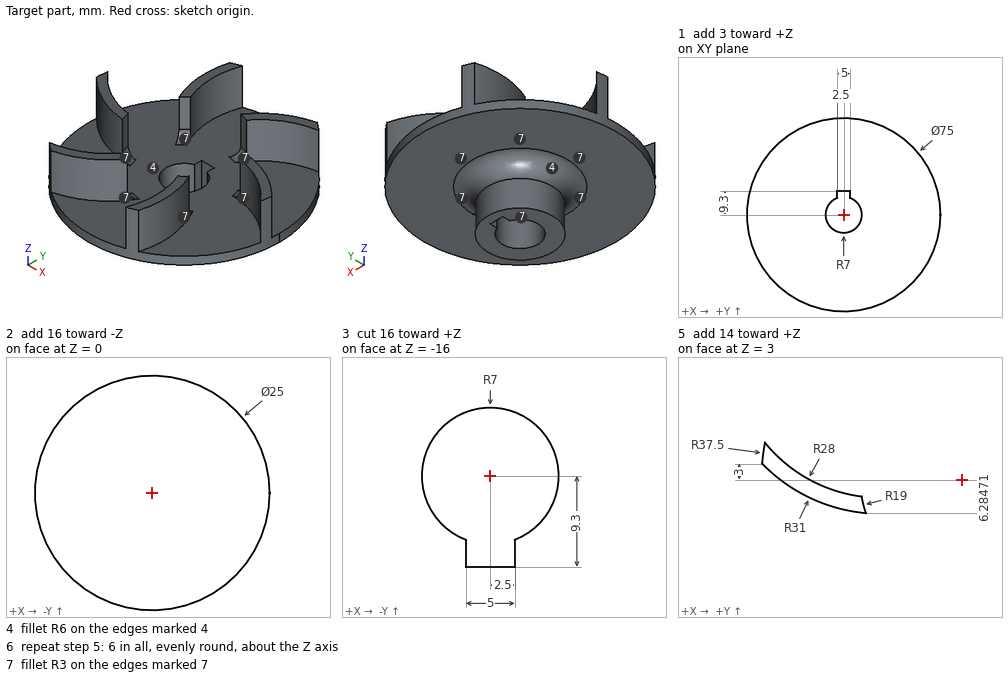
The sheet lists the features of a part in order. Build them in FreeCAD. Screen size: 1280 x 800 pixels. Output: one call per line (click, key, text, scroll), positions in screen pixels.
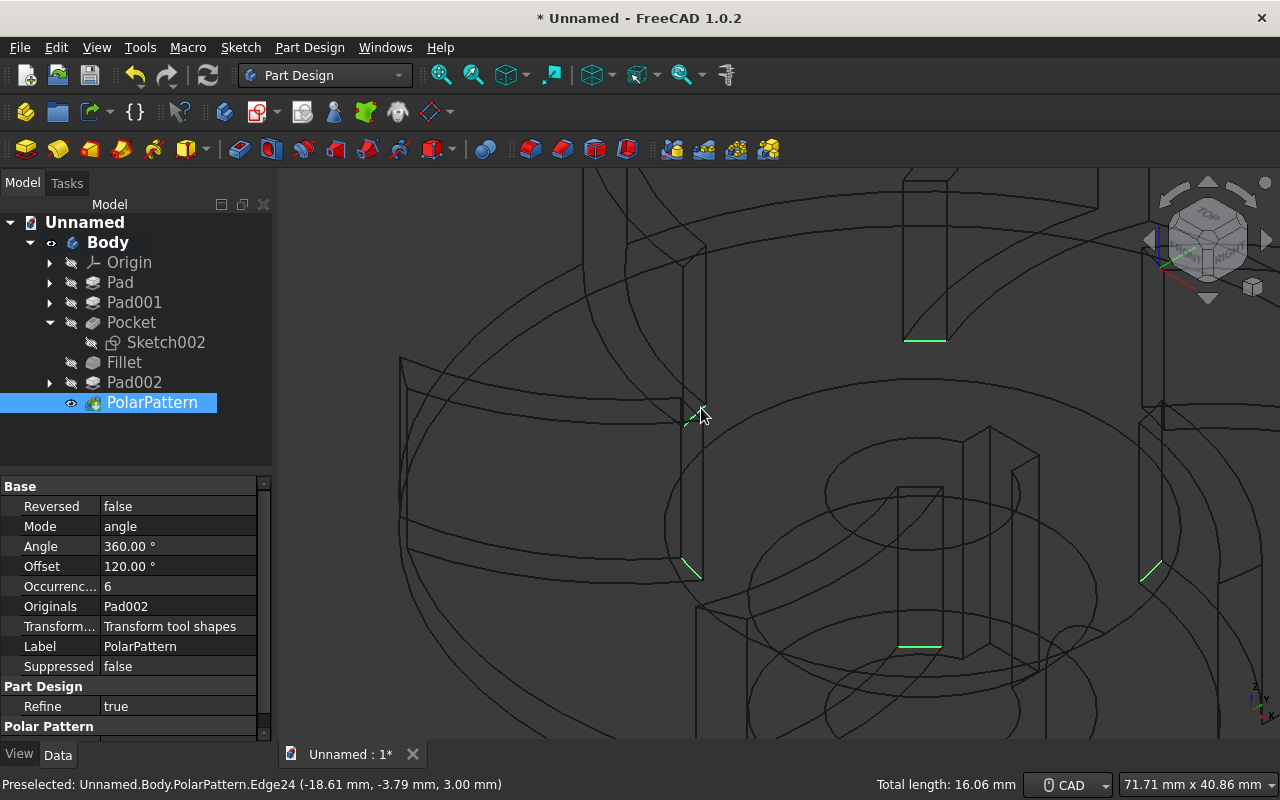
key(v)
key(f)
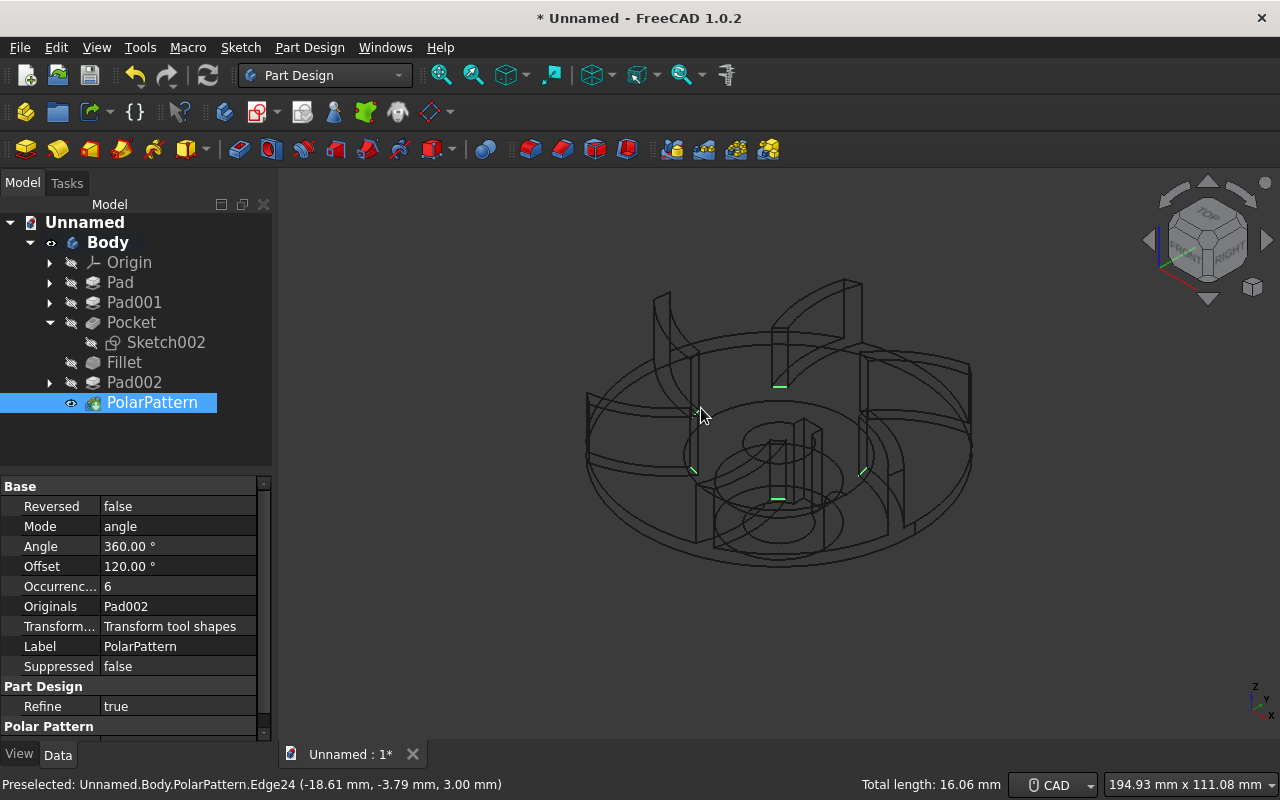
key(2)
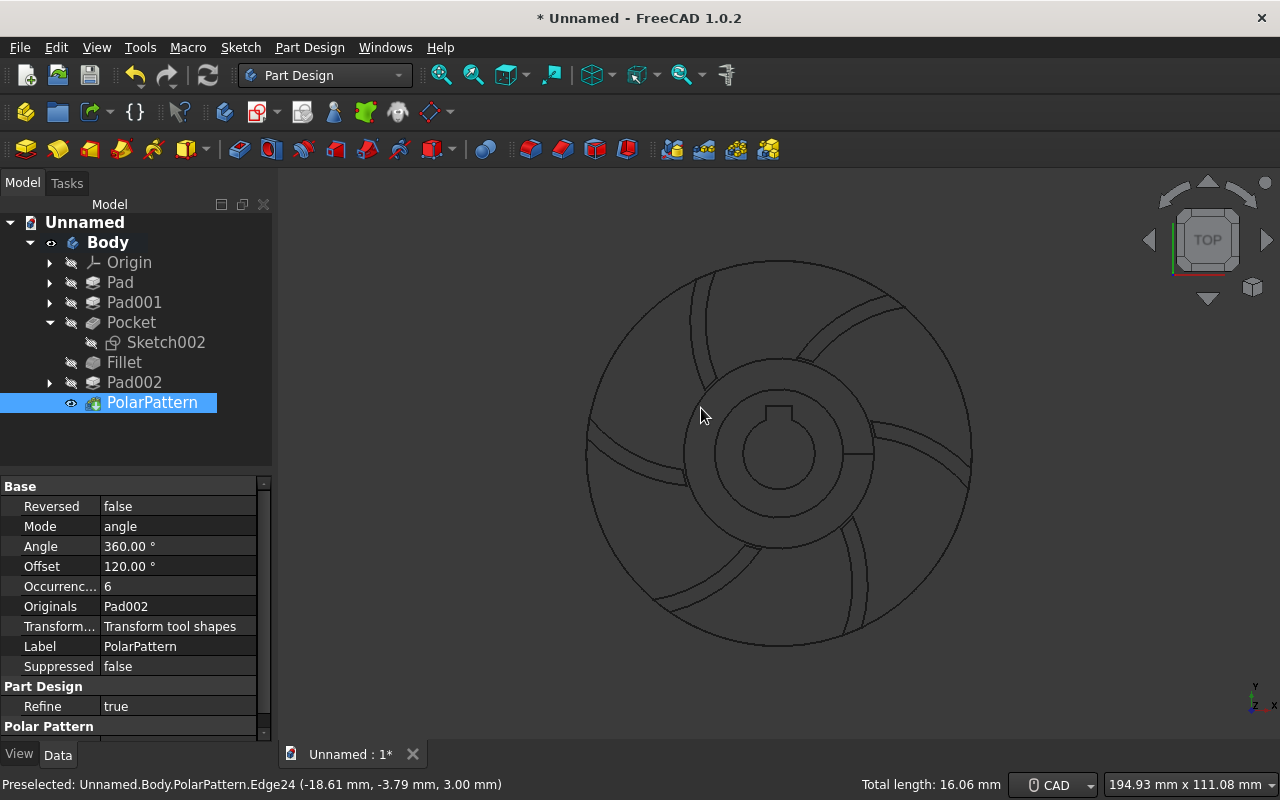
scroll(805, 358, up, 5)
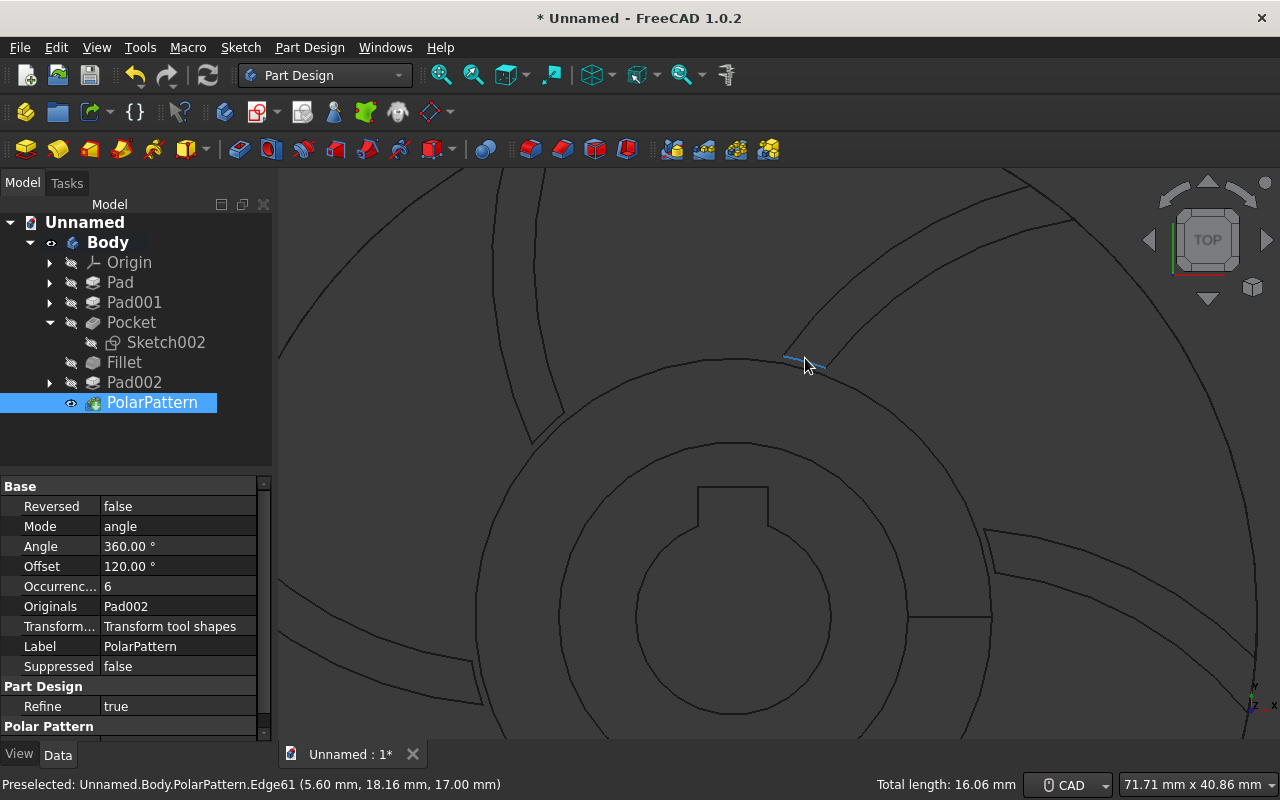
key(v)
key(f)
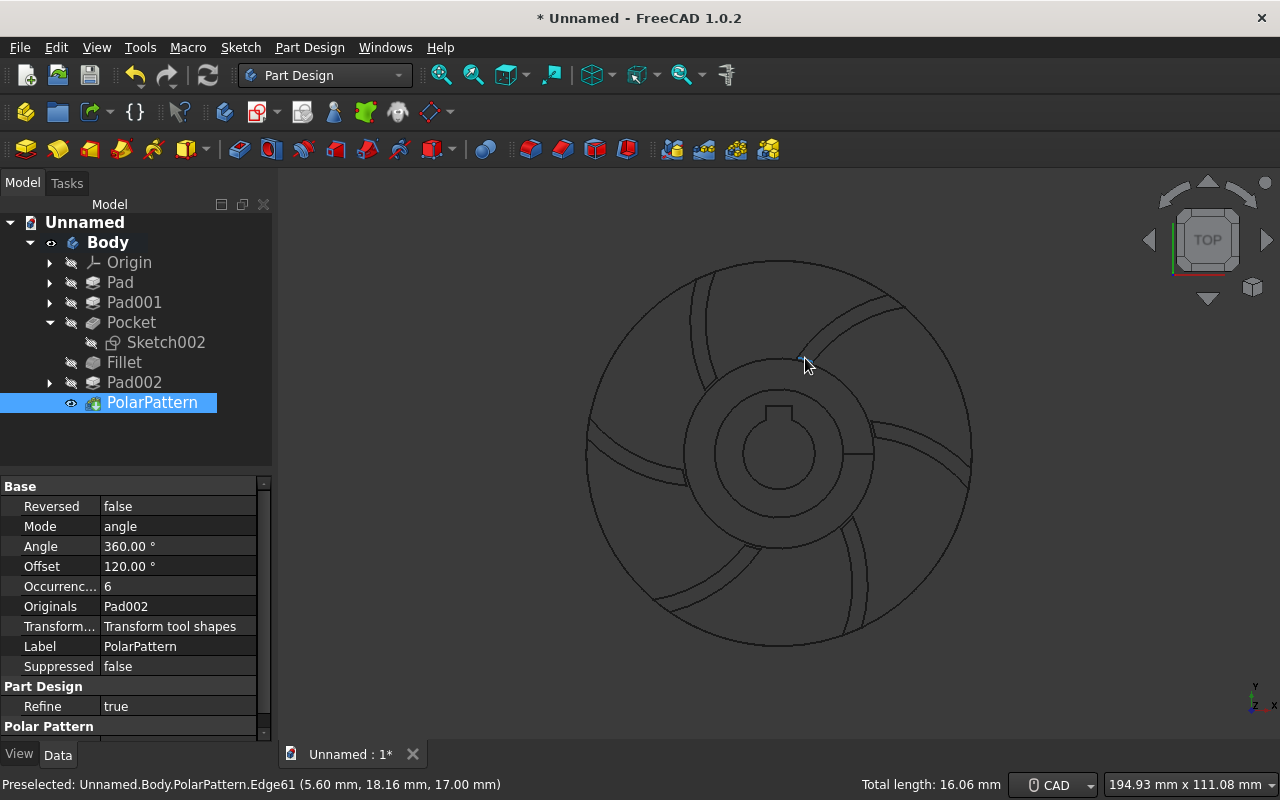
key(1)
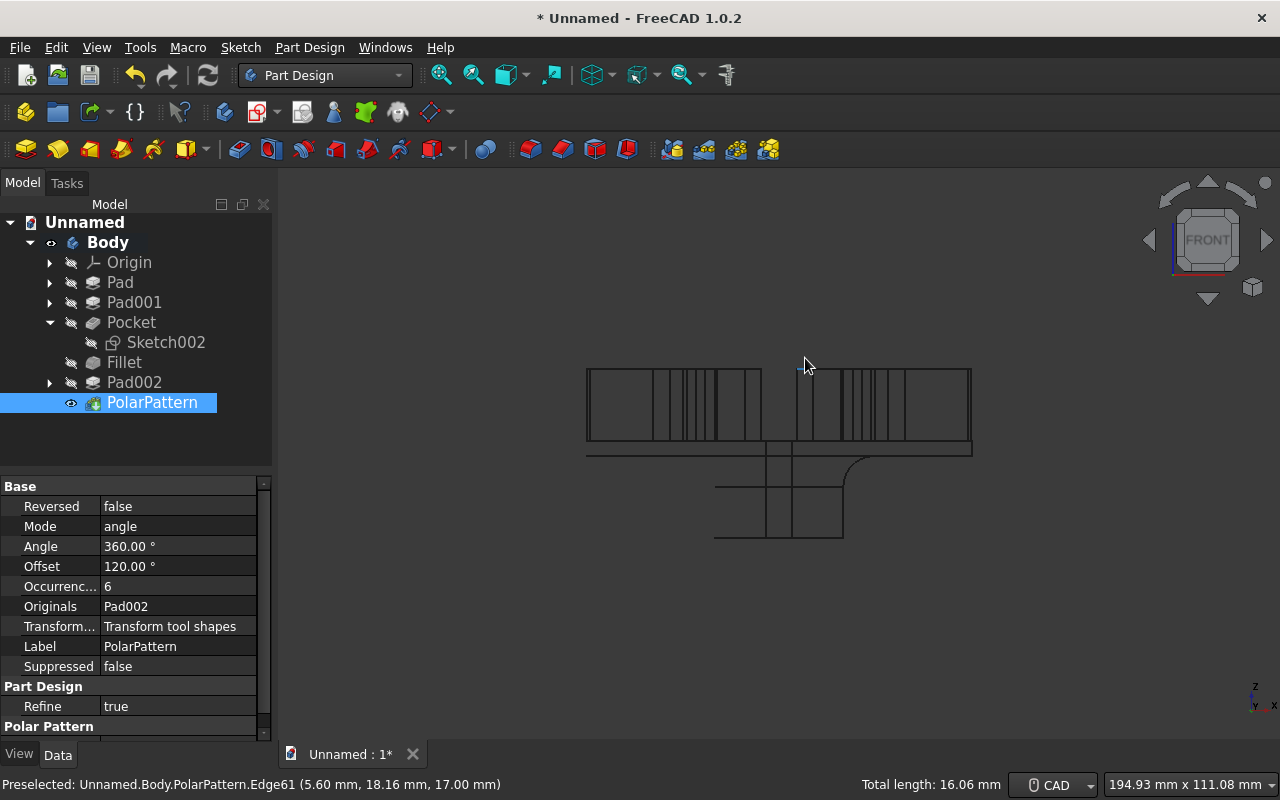
key(v)
key(f)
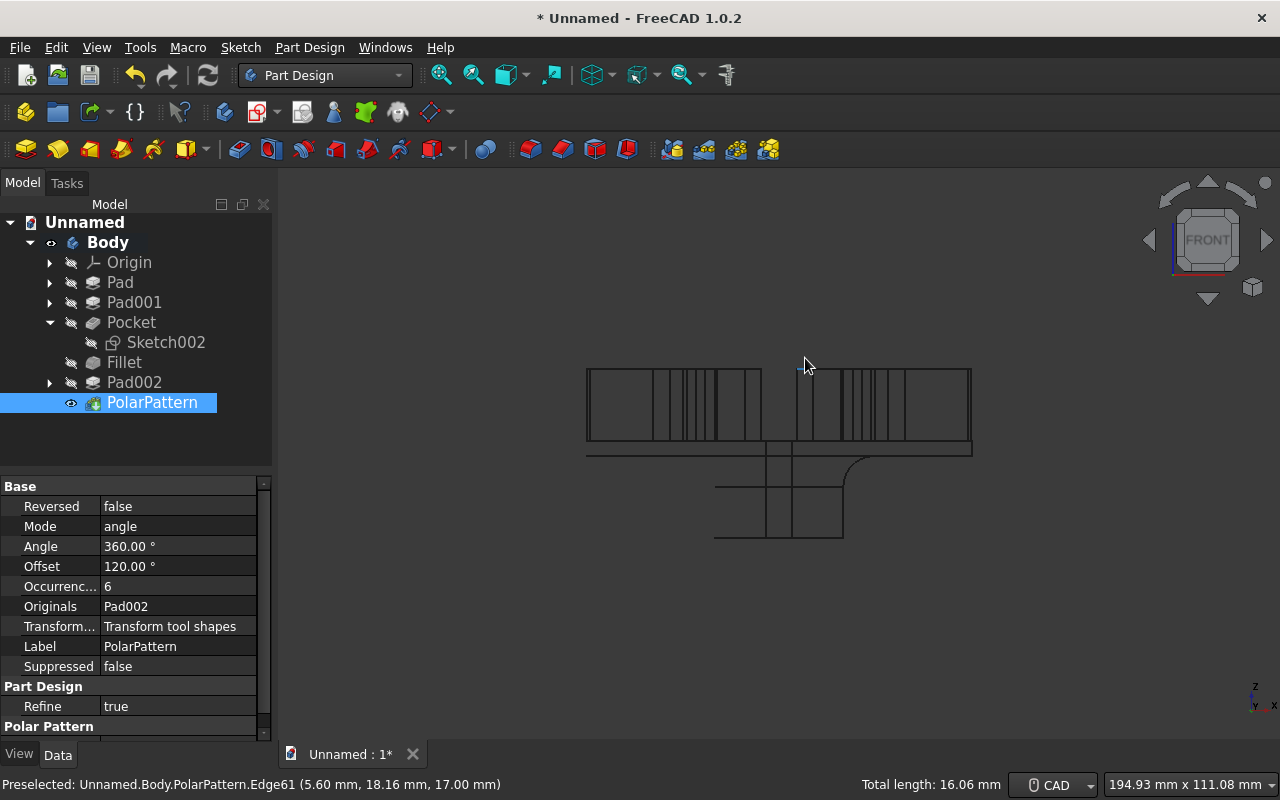
scroll(805, 440, up, 5)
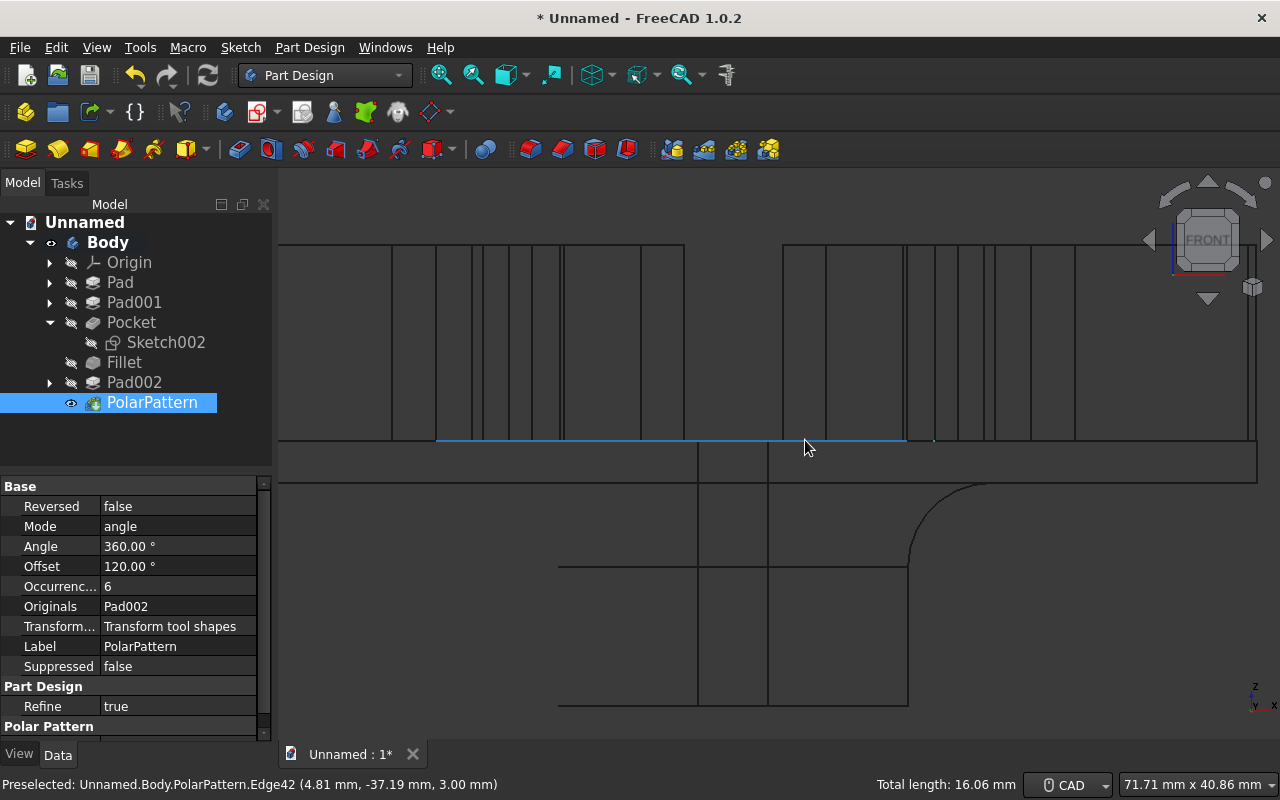
key(v)
key(f)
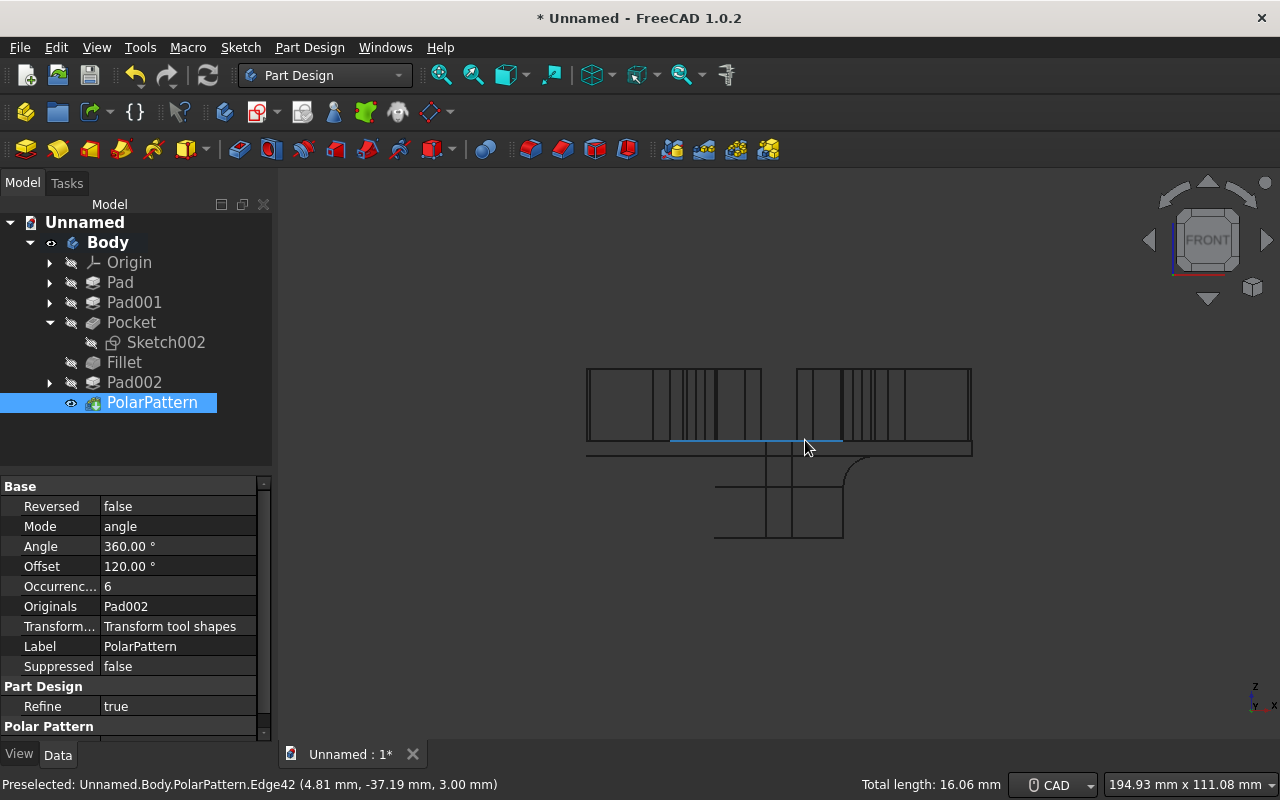
key(3)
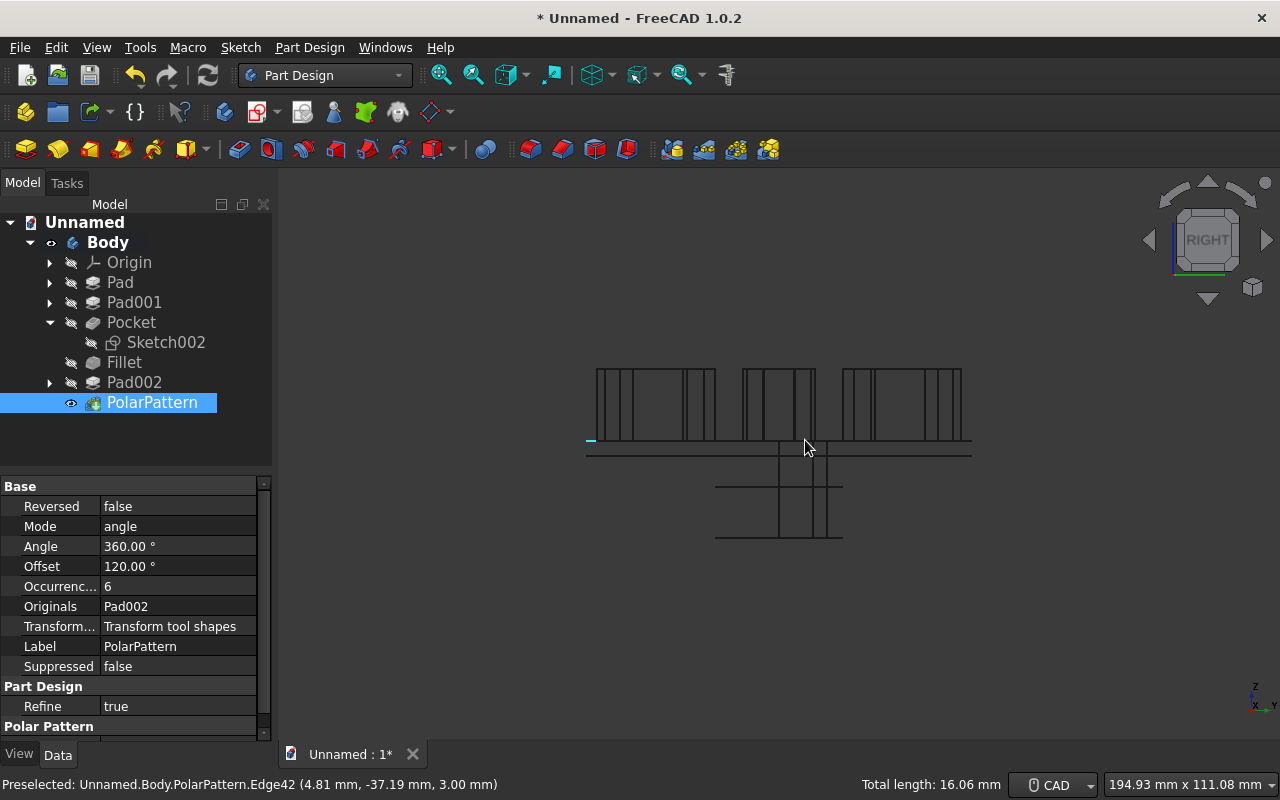
key(v)
key(f)